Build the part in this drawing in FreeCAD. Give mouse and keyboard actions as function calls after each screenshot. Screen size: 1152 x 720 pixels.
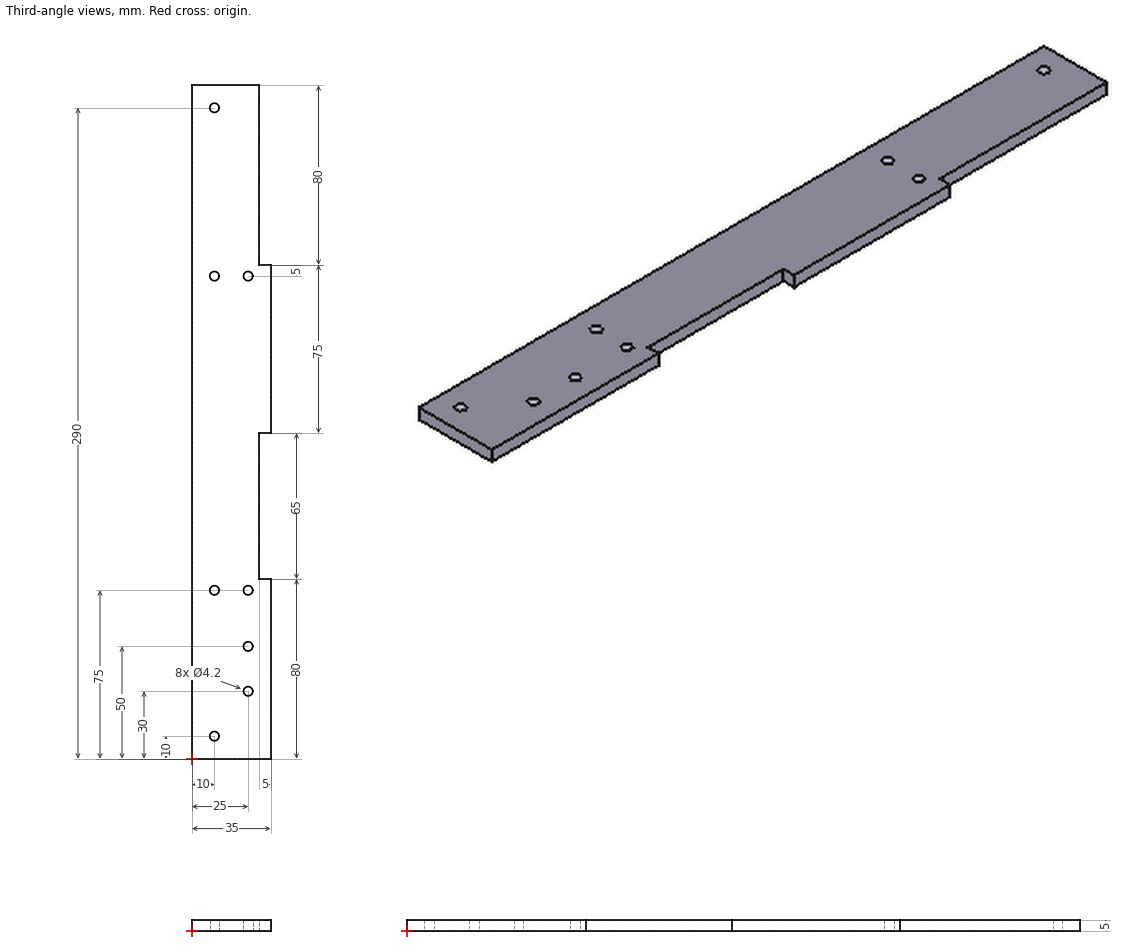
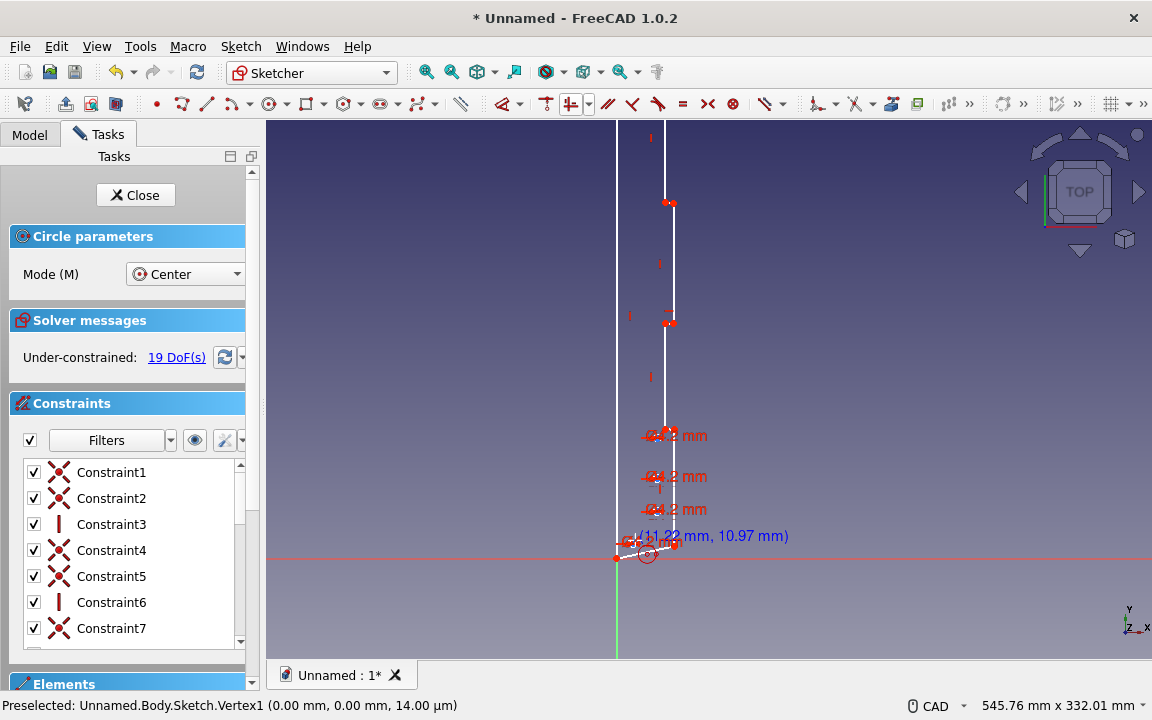
scroll(633, 437, up, 10)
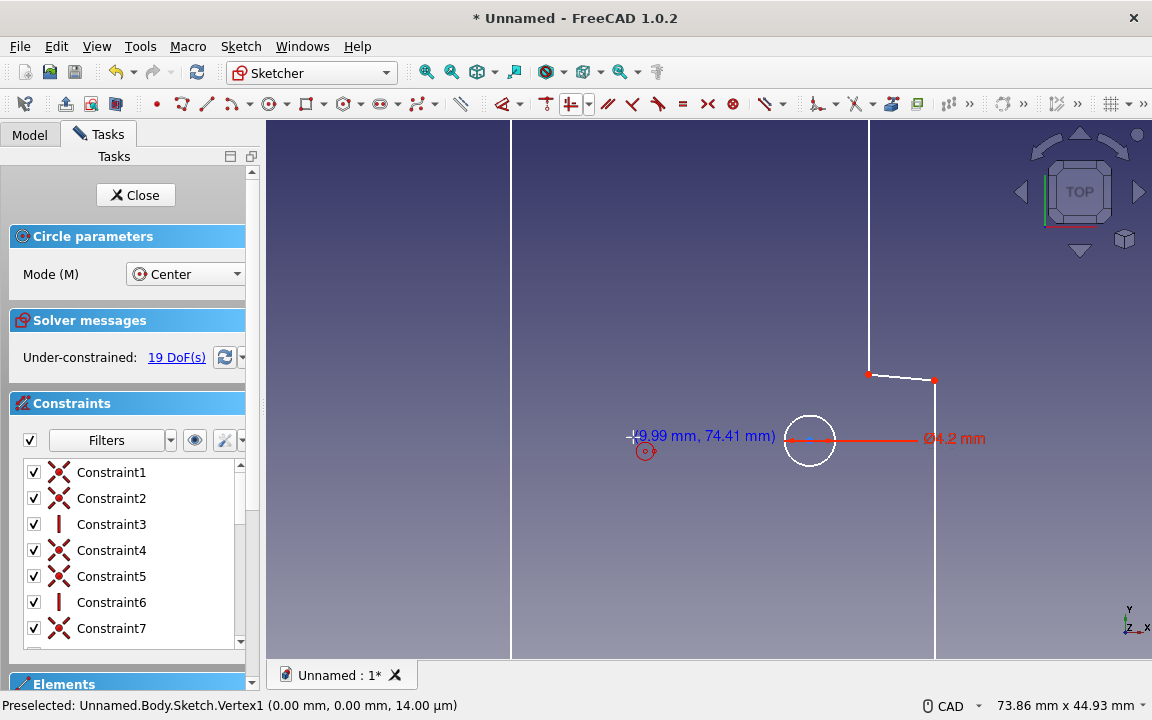
scroll(633, 475, down, 12)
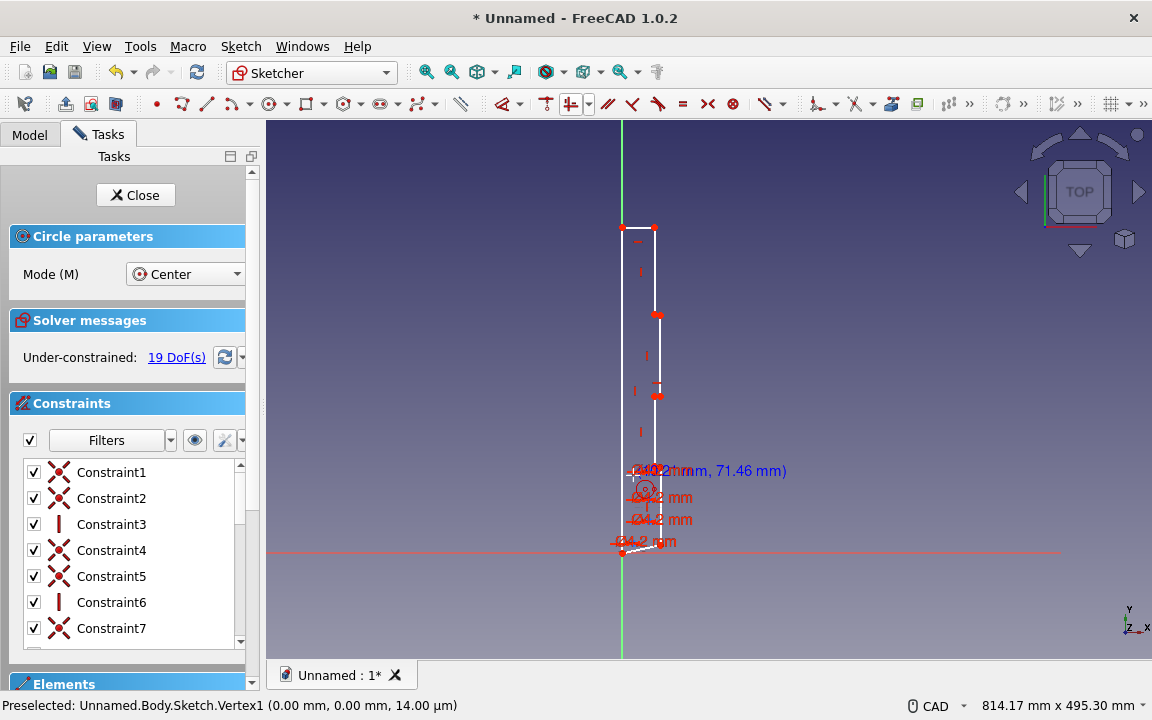
scroll(633, 472, up, 2)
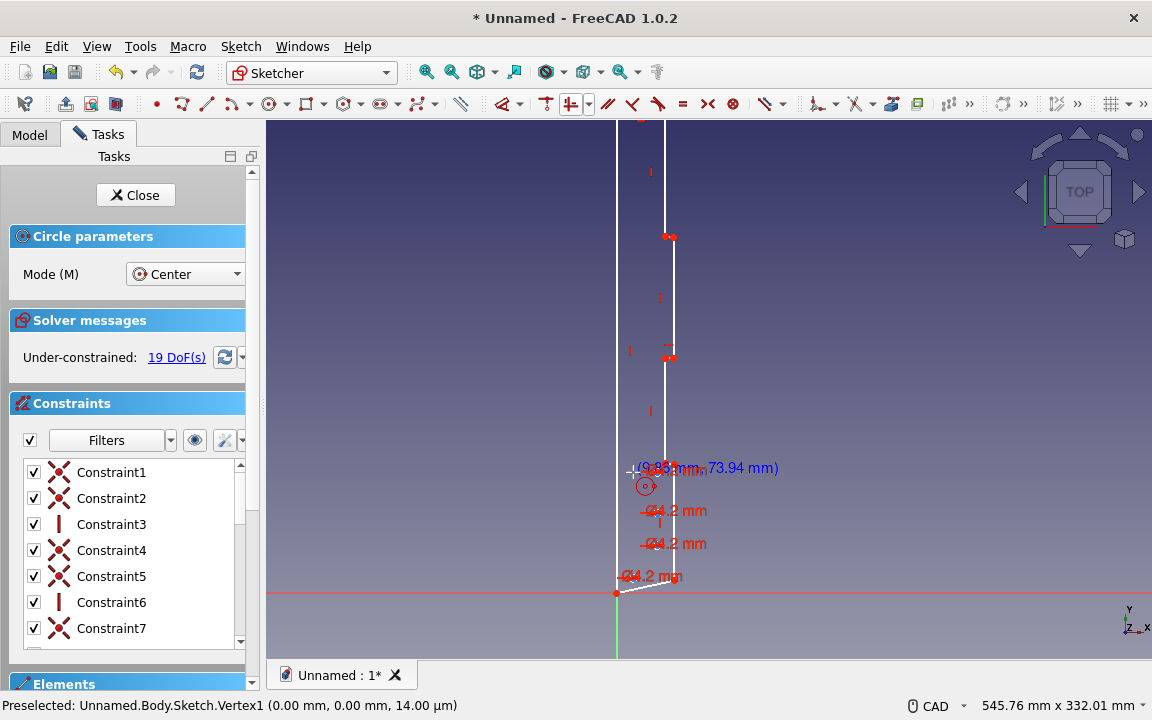
click(633, 471)
move(635, 469)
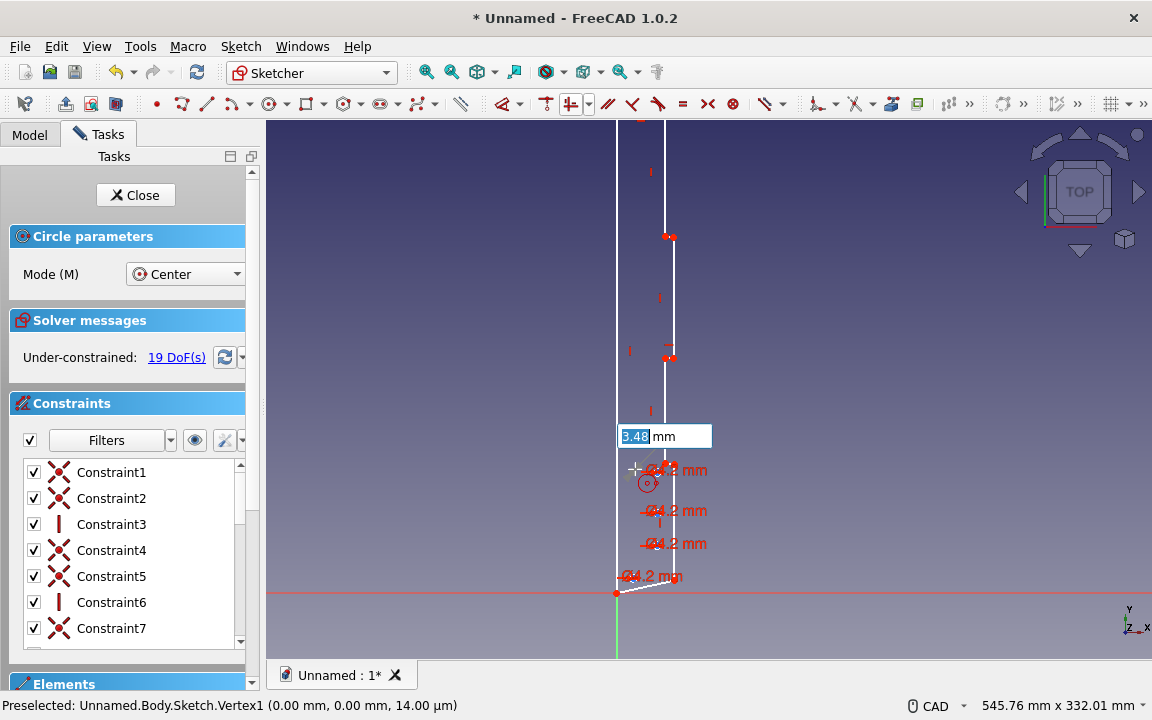
text(4.2)
key(Return)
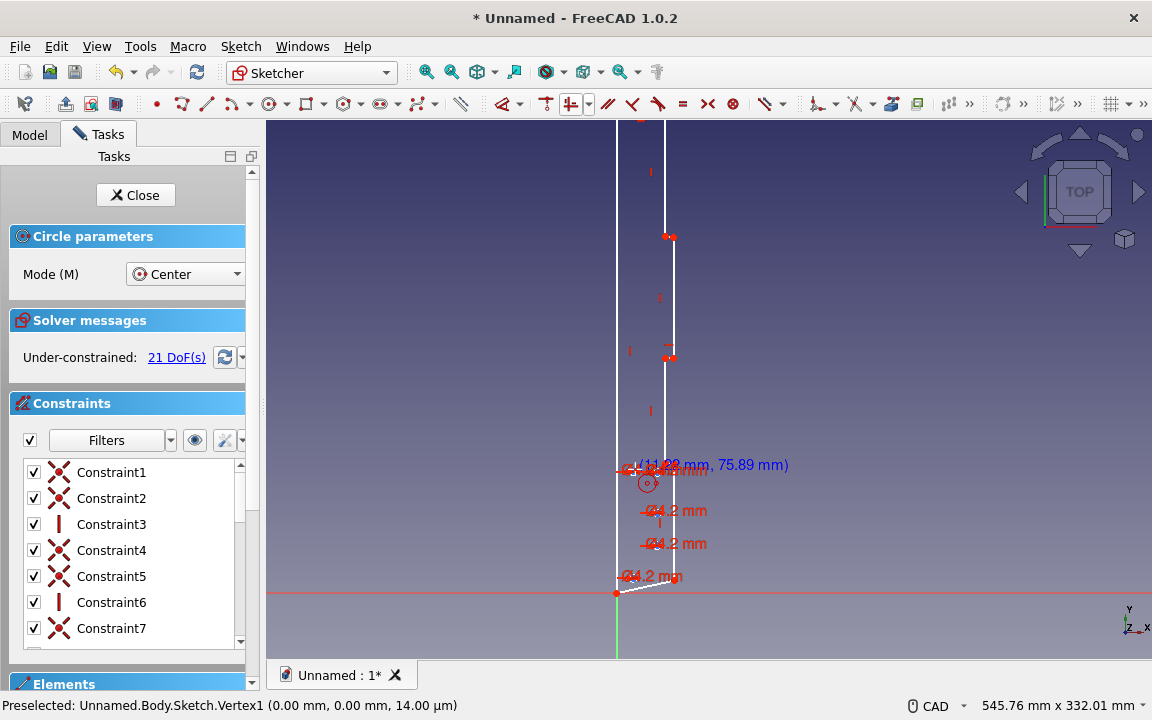
scroll(657, 244, up, 10)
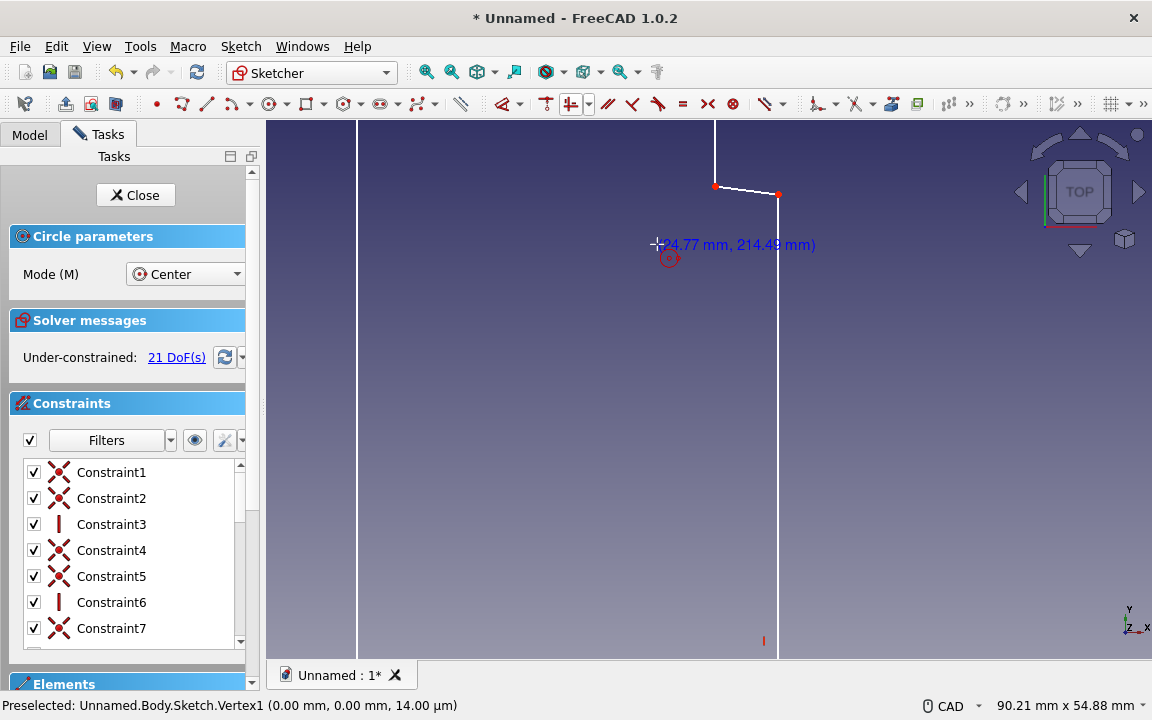
scroll(648, 326, down, 12)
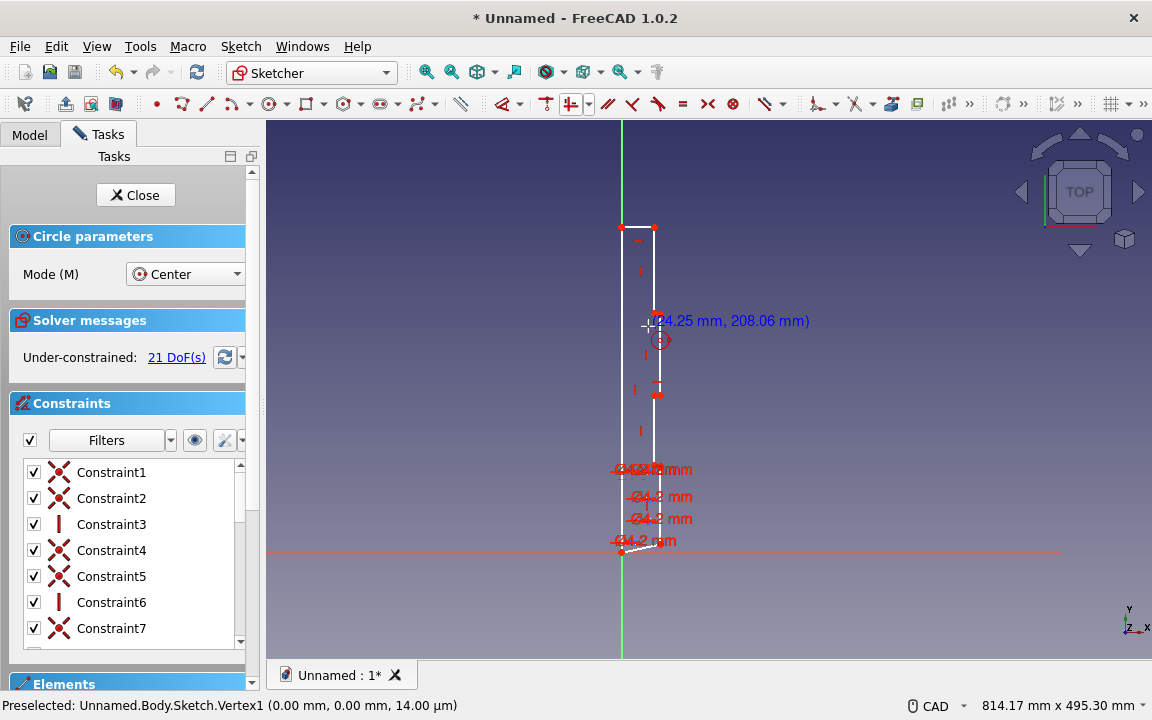
scroll(649, 319, up, 4)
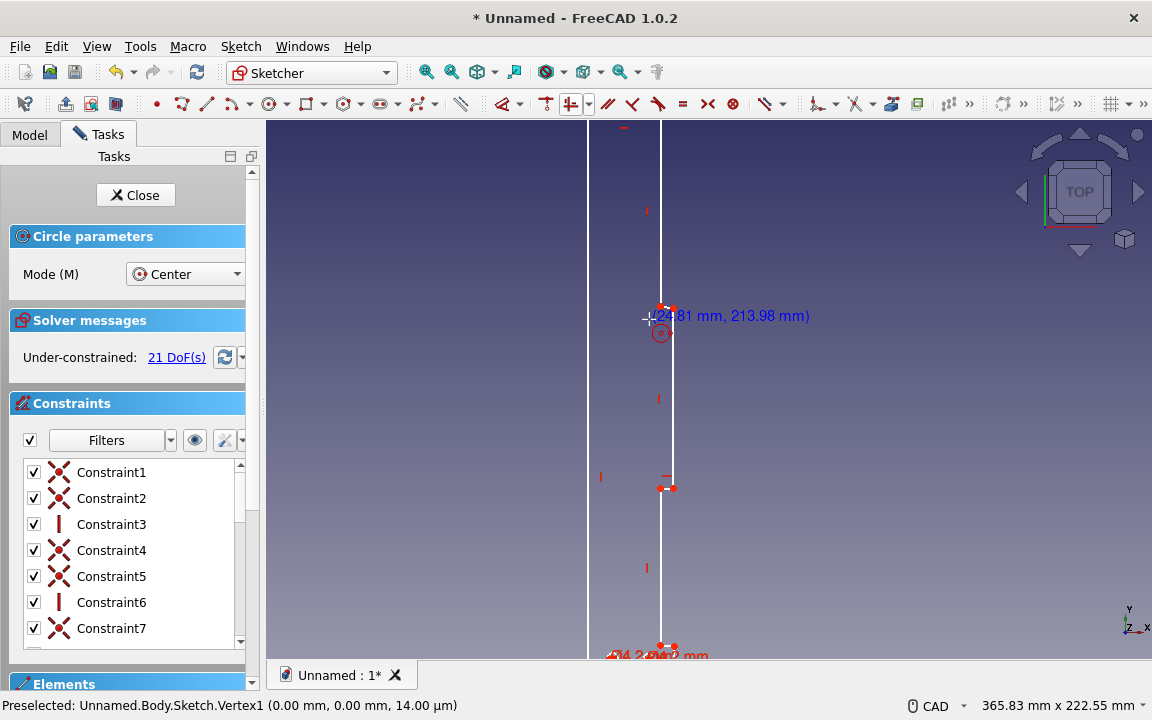
click(649, 318)
move(645, 315)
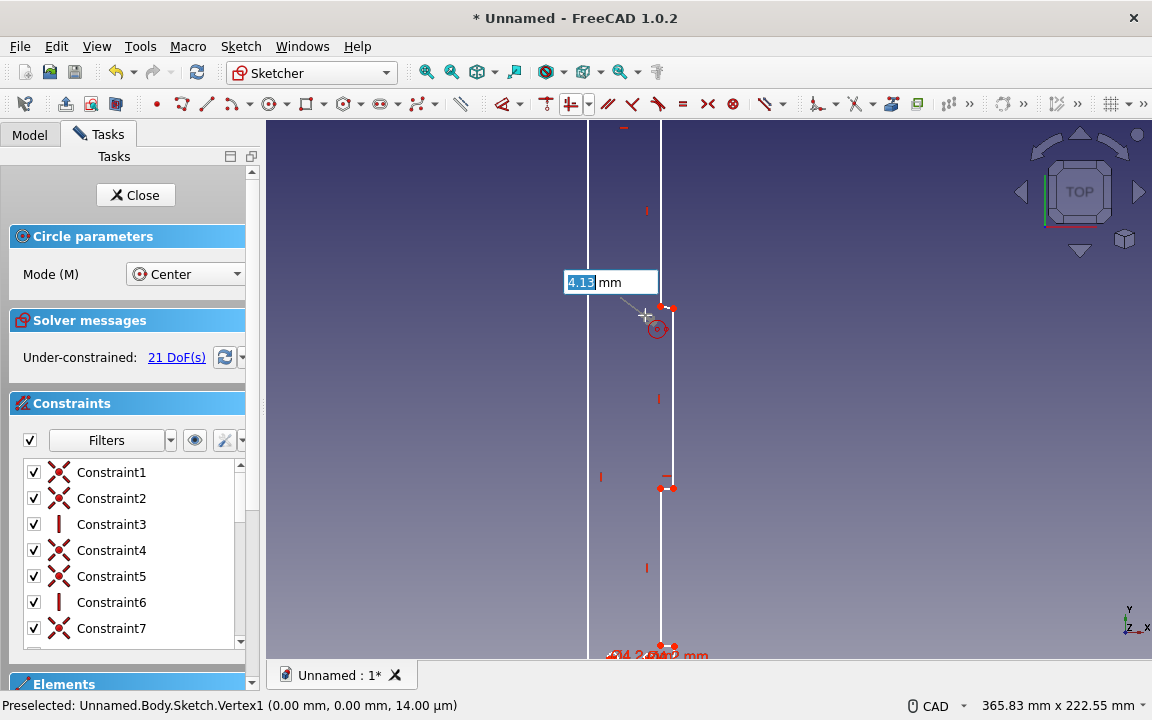
text(4.2)
key(Return)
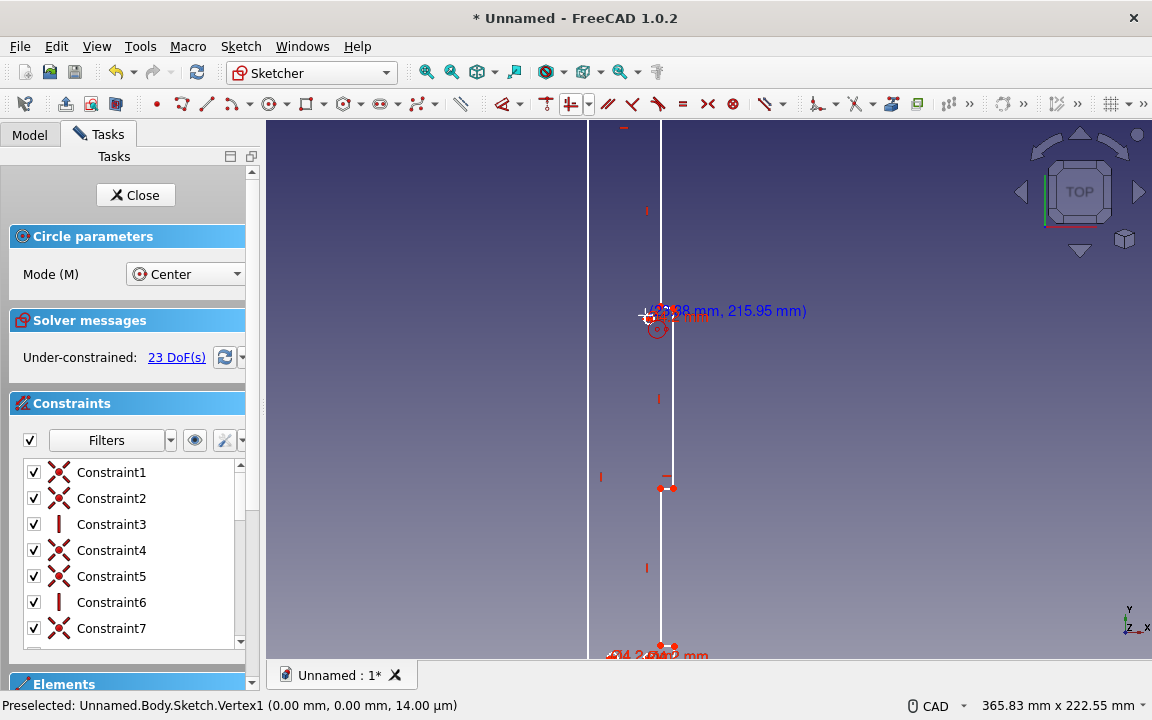
scroll(613, 318, up, 8)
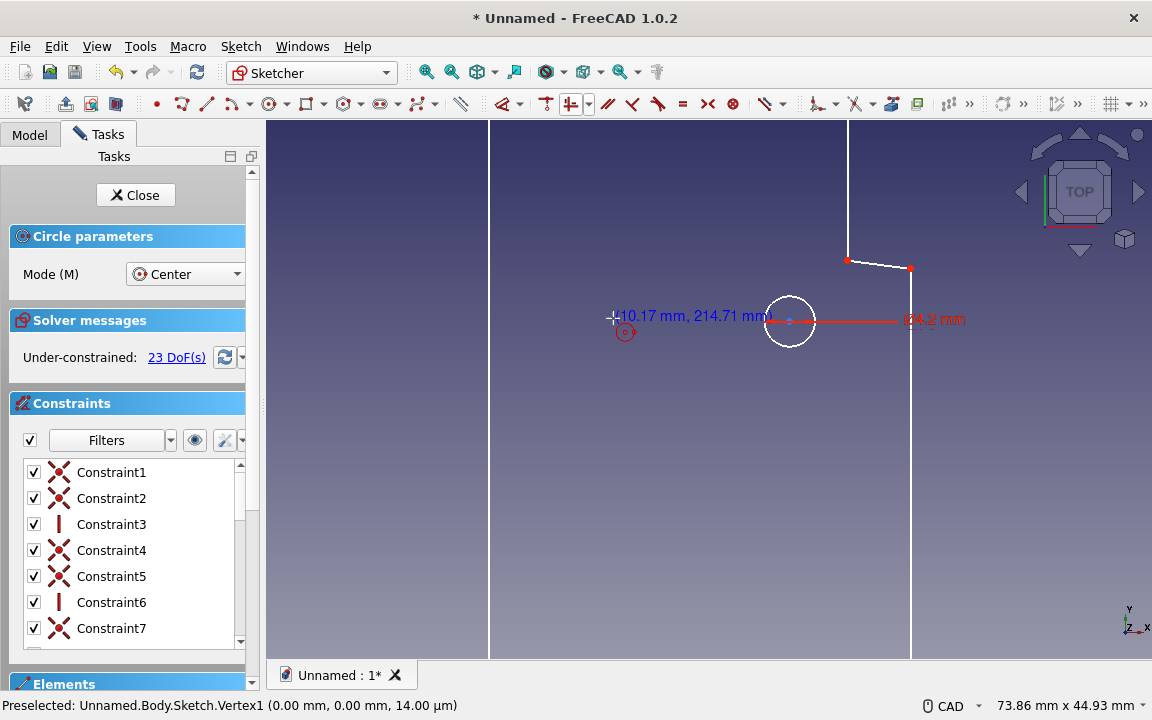
scroll(635, 319, down, 12)